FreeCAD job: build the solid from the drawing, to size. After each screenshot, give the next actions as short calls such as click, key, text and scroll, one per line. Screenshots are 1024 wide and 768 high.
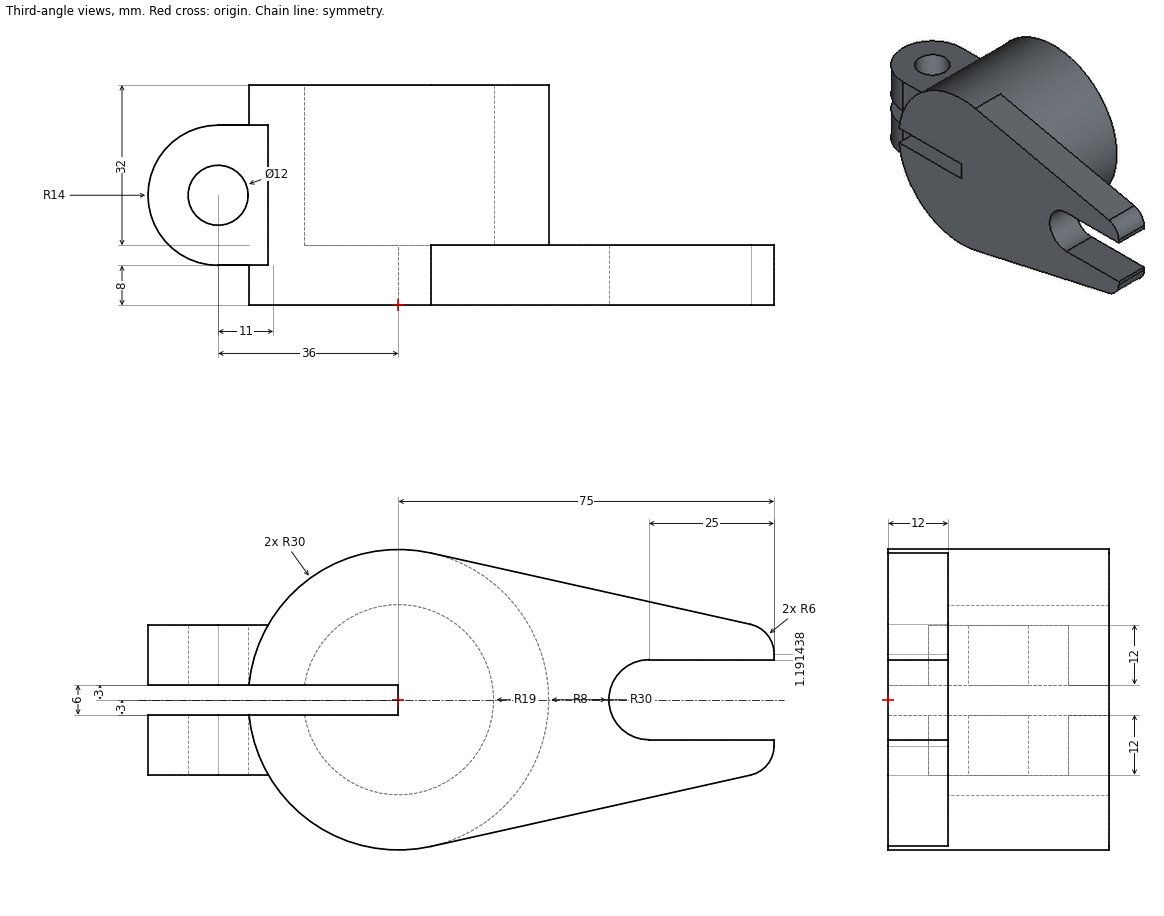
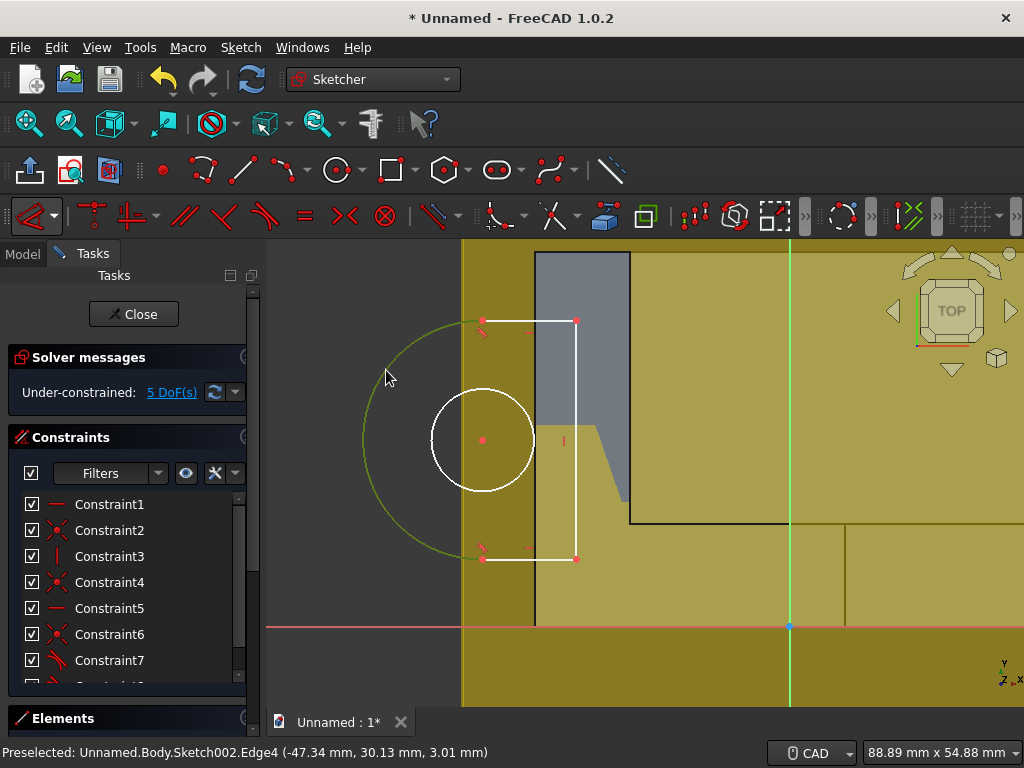
key(k)
key(r)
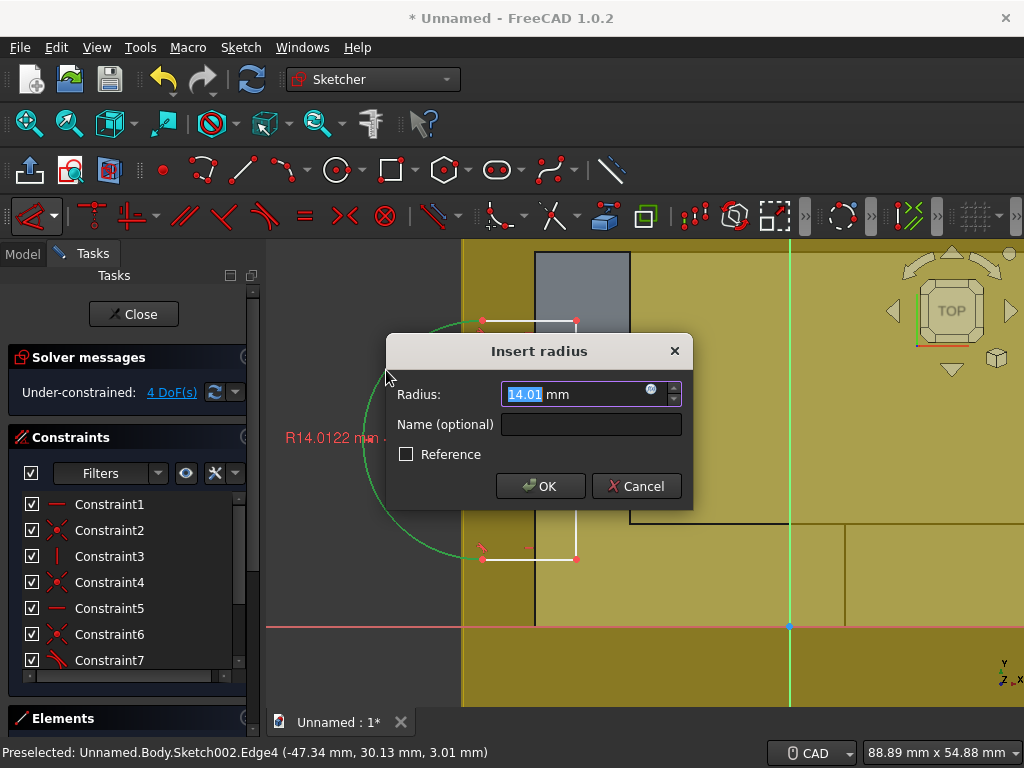
text(14)
key(Return)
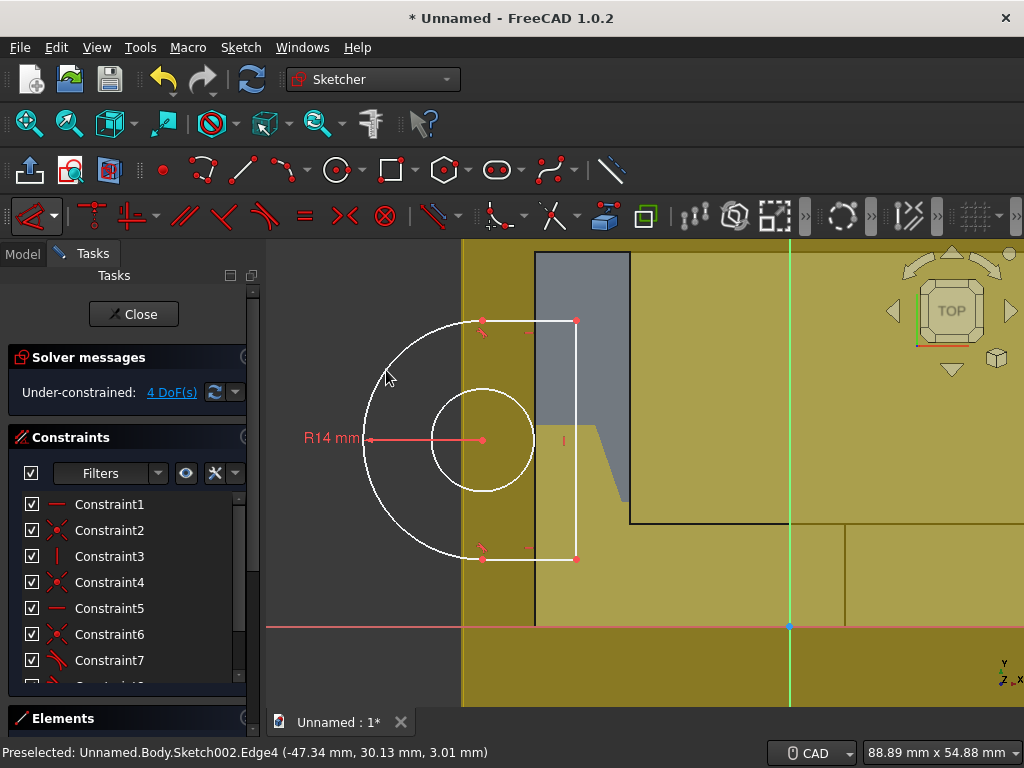
click(519, 404)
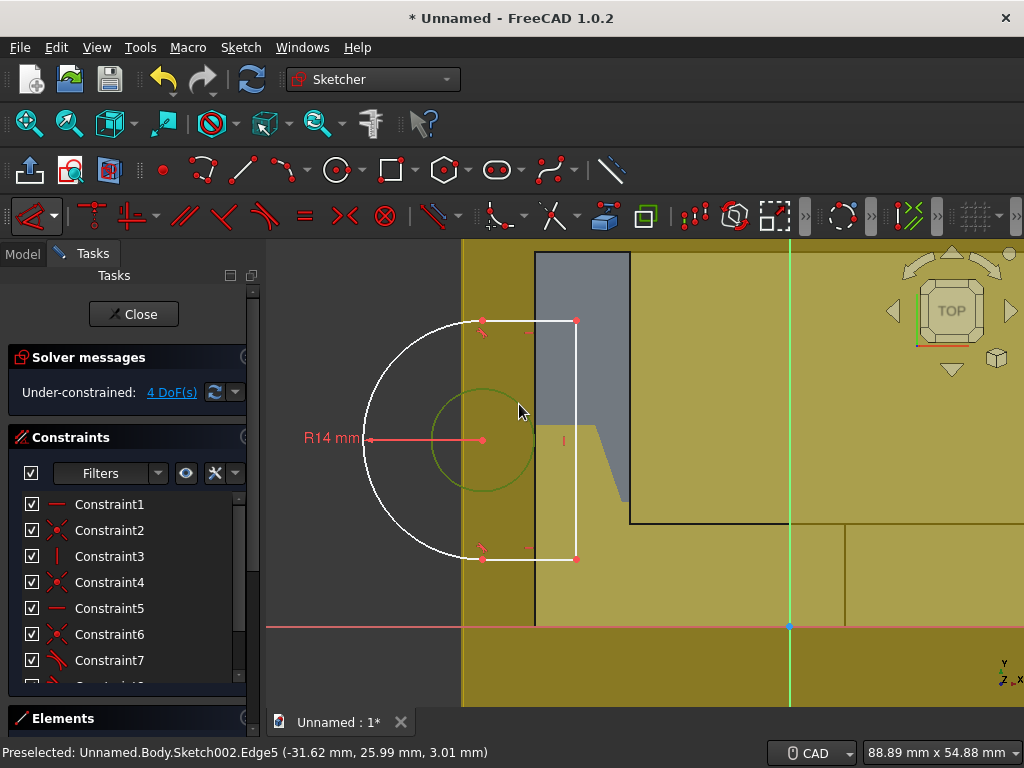
click(56, 216)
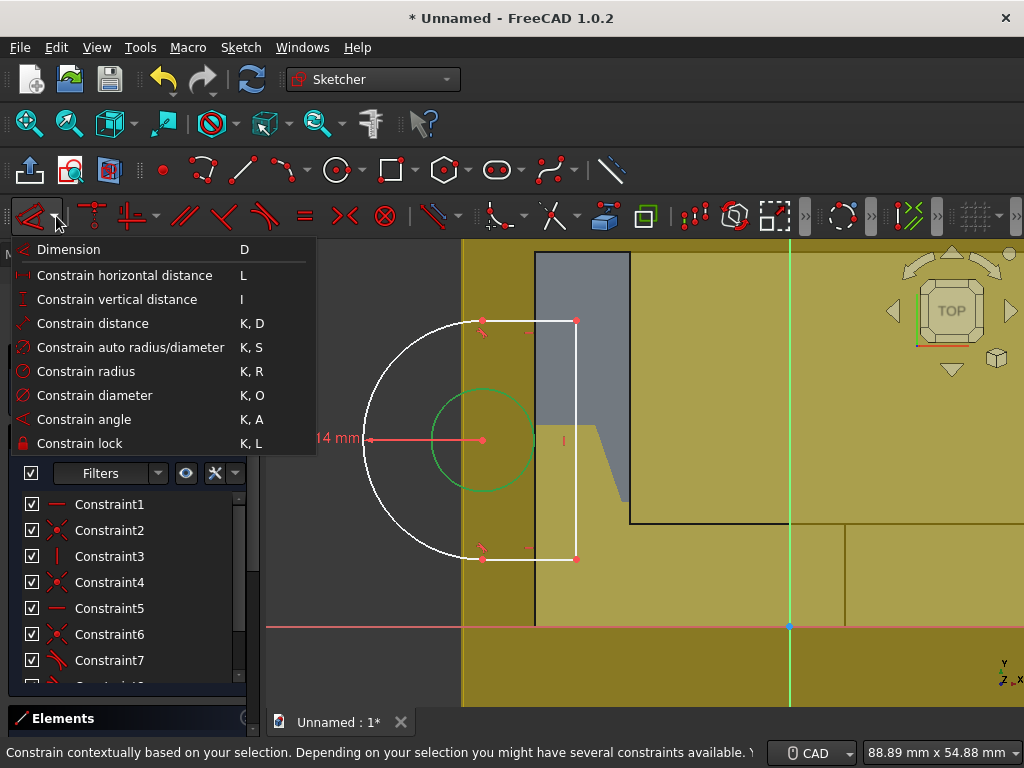
click(164, 395)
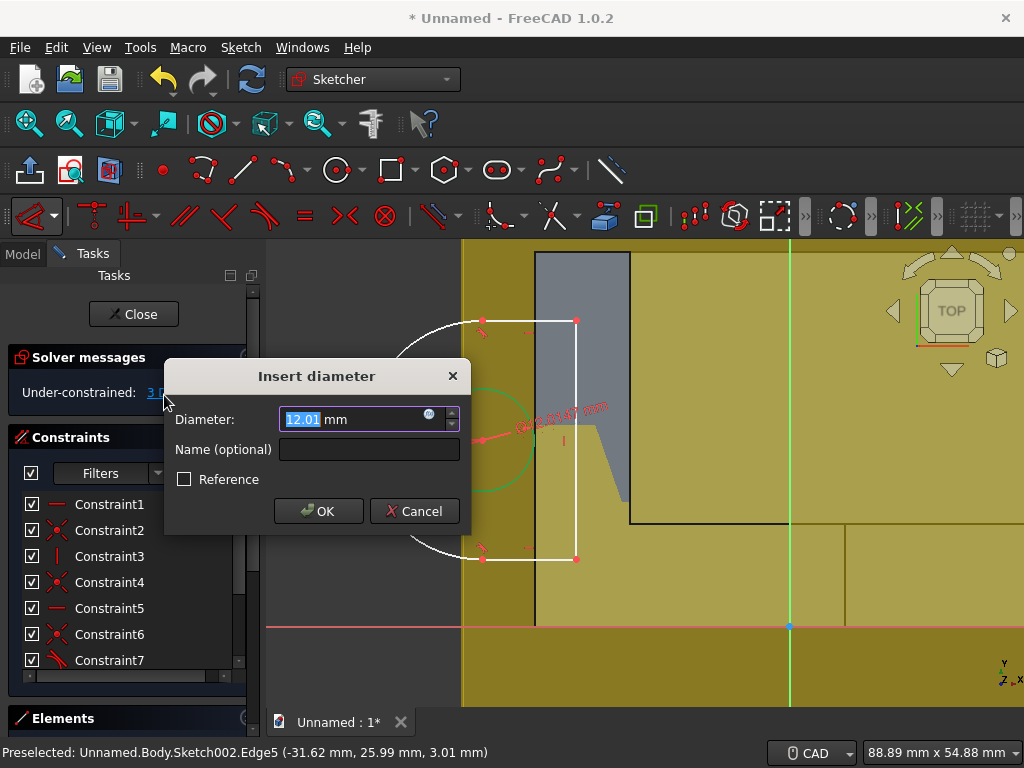
text(12)
key(Return)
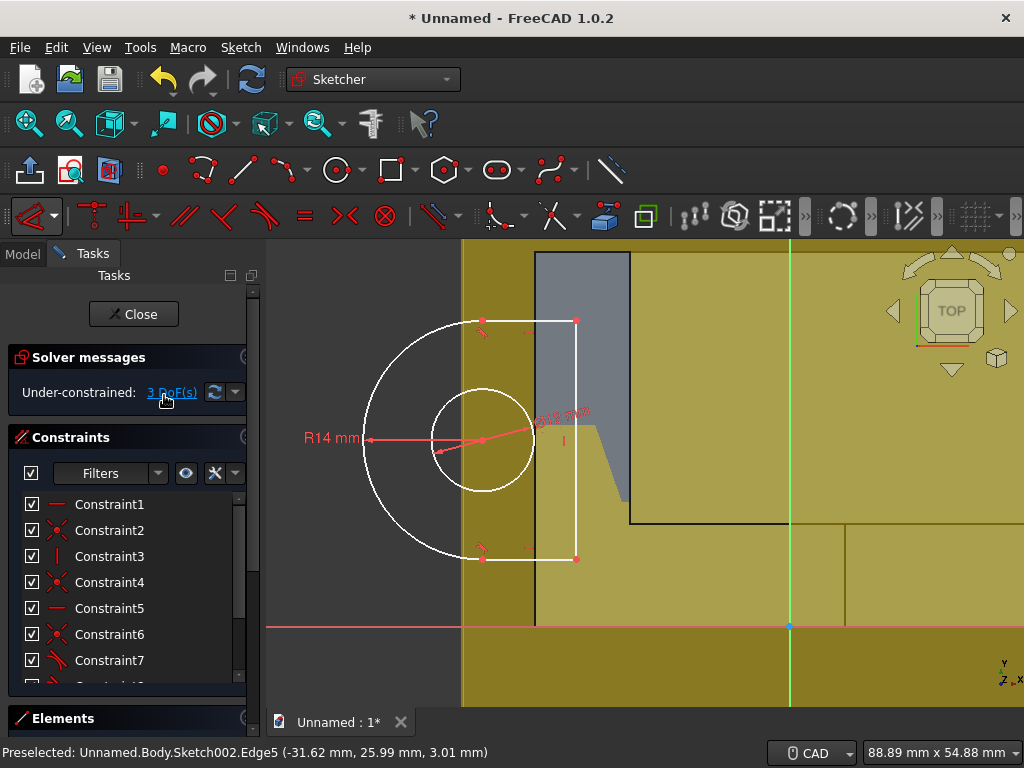
click(511, 560)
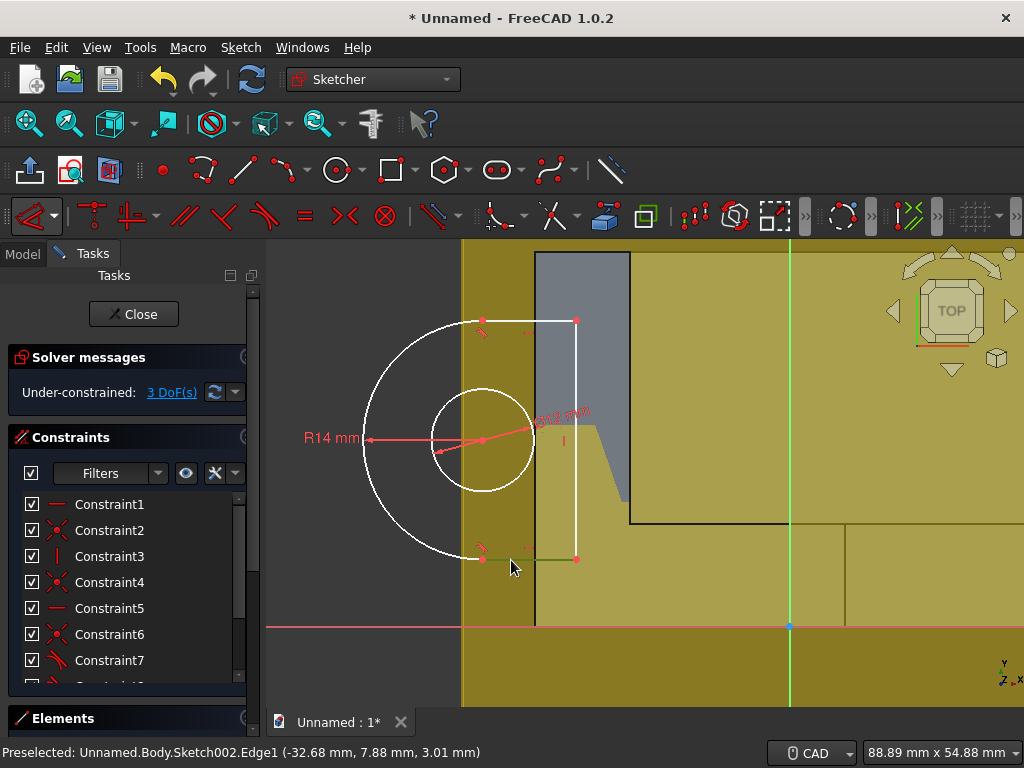
key(l)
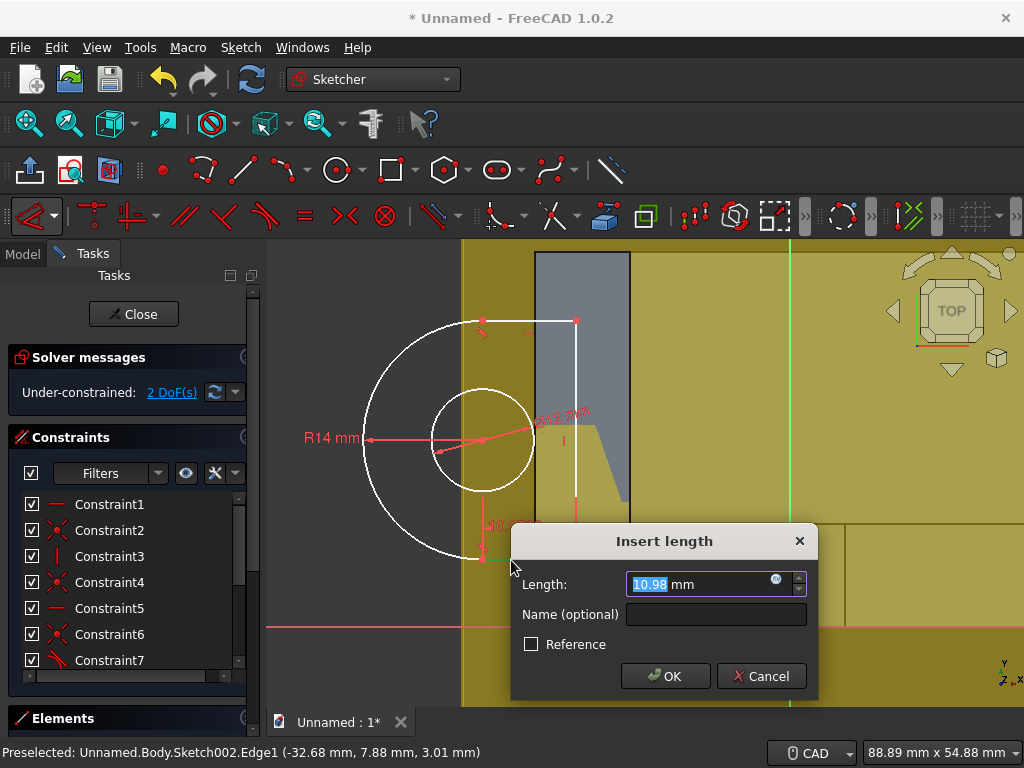
text(11)
key(Return)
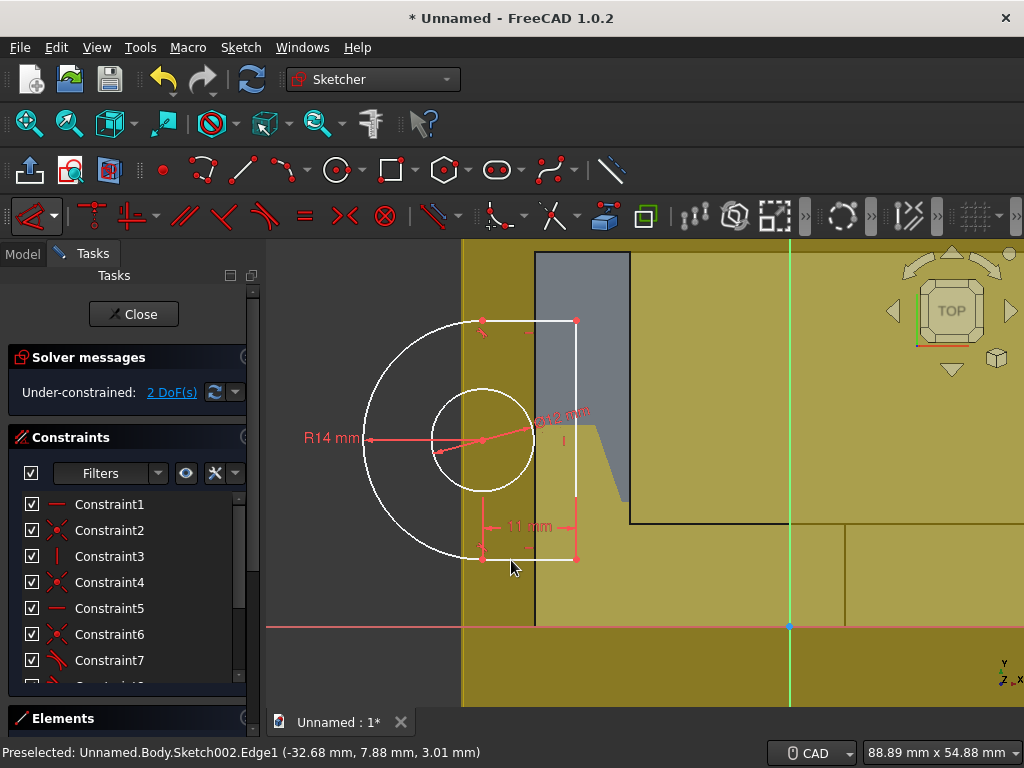
click(483, 560)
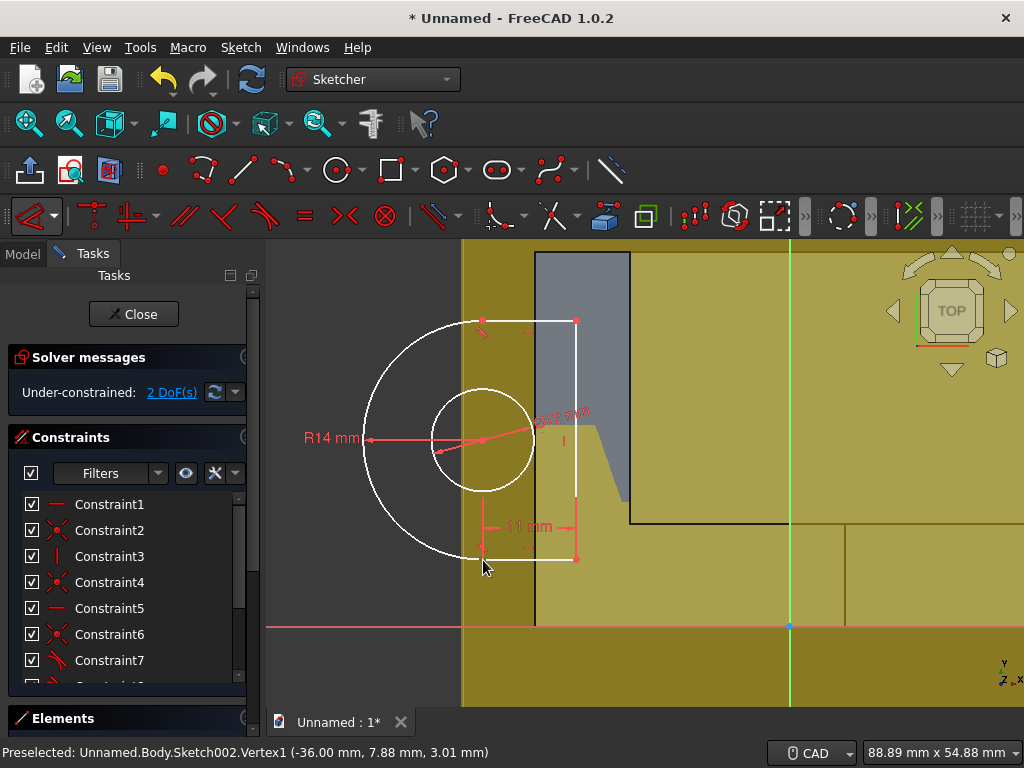
click(56, 216)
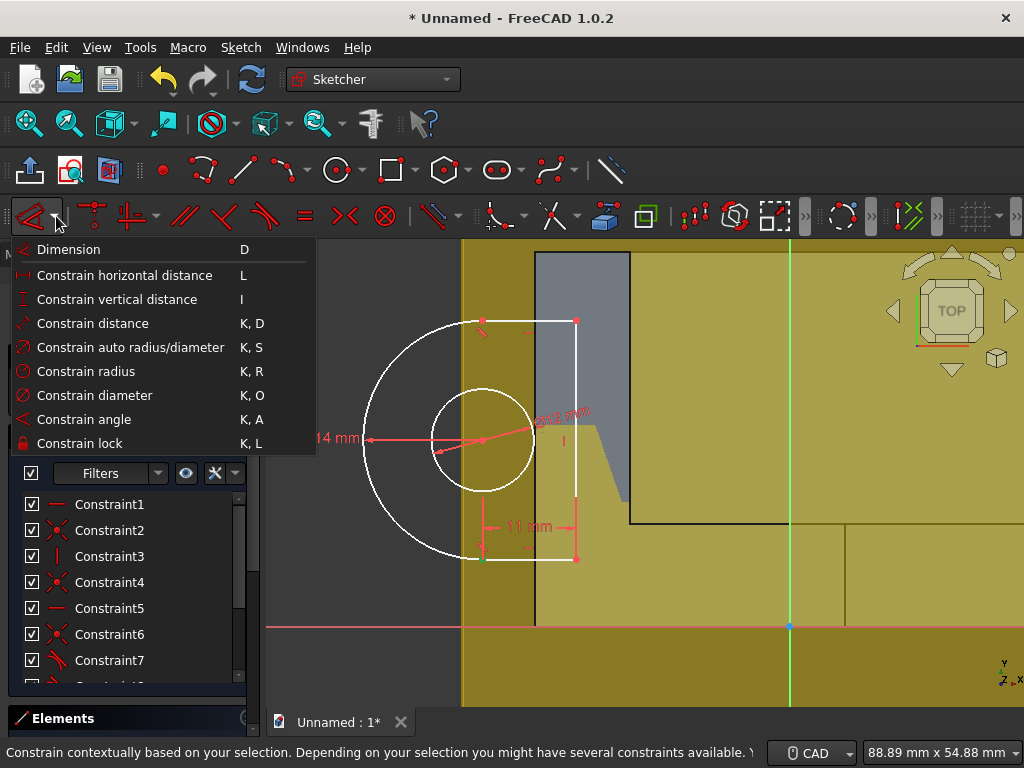
click(164, 299)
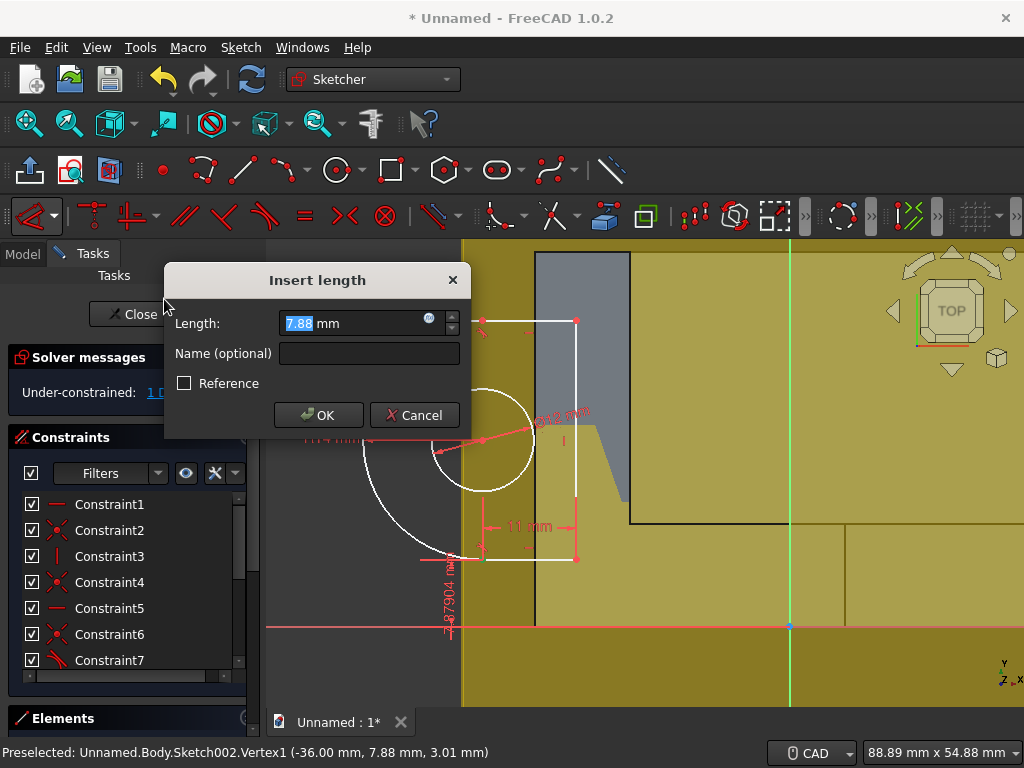
text(8)
key(Return)